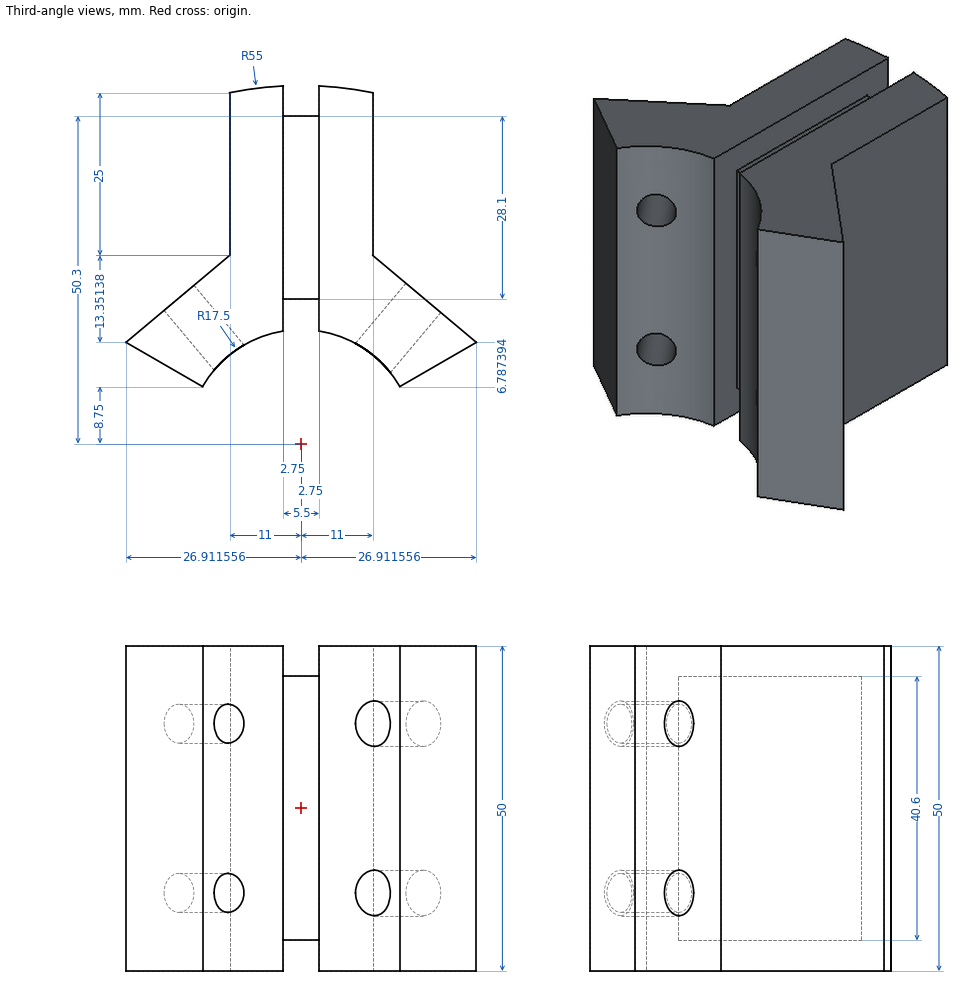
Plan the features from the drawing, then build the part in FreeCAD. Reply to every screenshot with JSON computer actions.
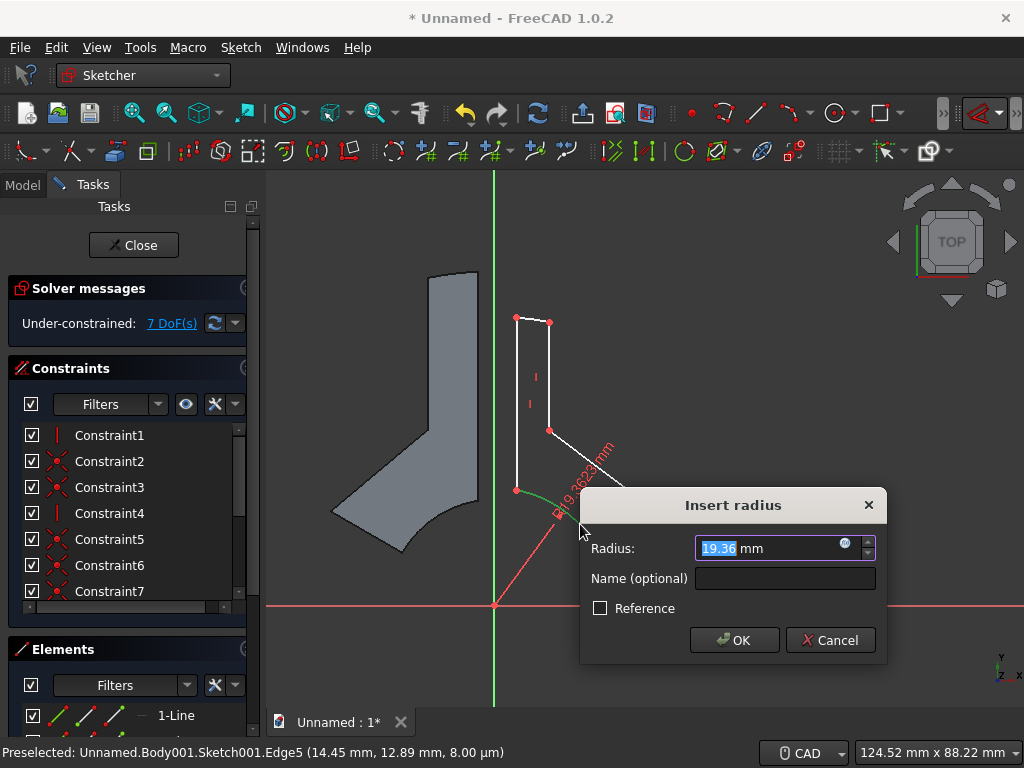
{"action": "type", "text": "17.5"}
{"action": "key", "text": "Return"}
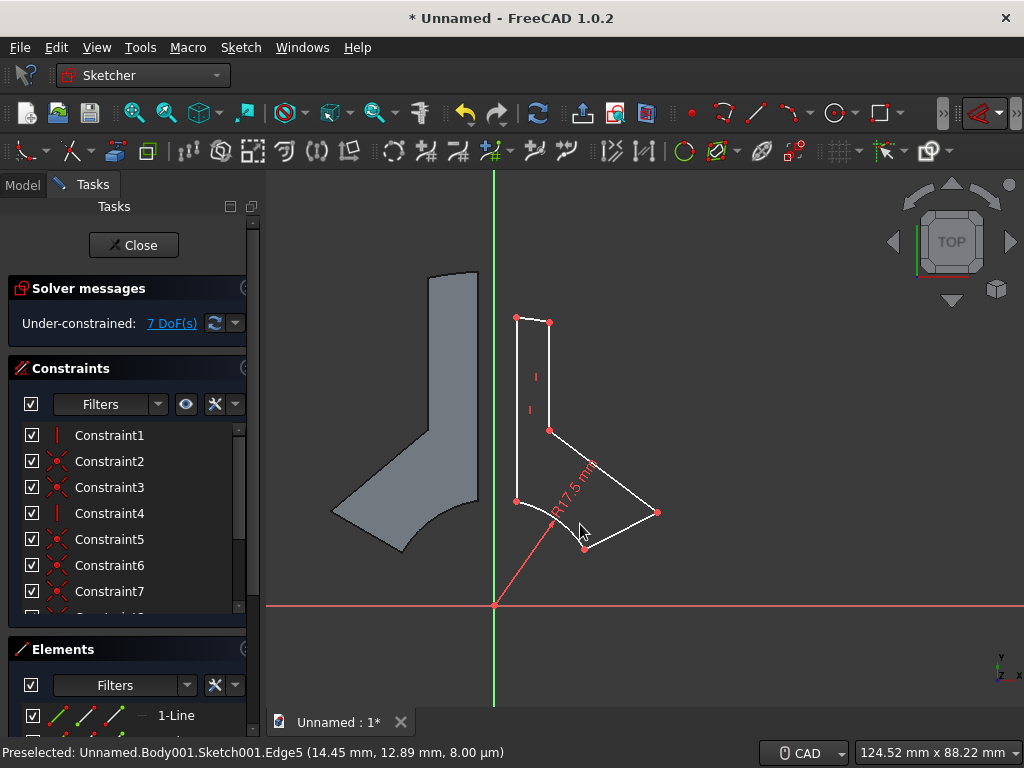
{"action": "scroll", "coordinate": [540, 320], "scroll_direction": "up", "scroll_amount": 2}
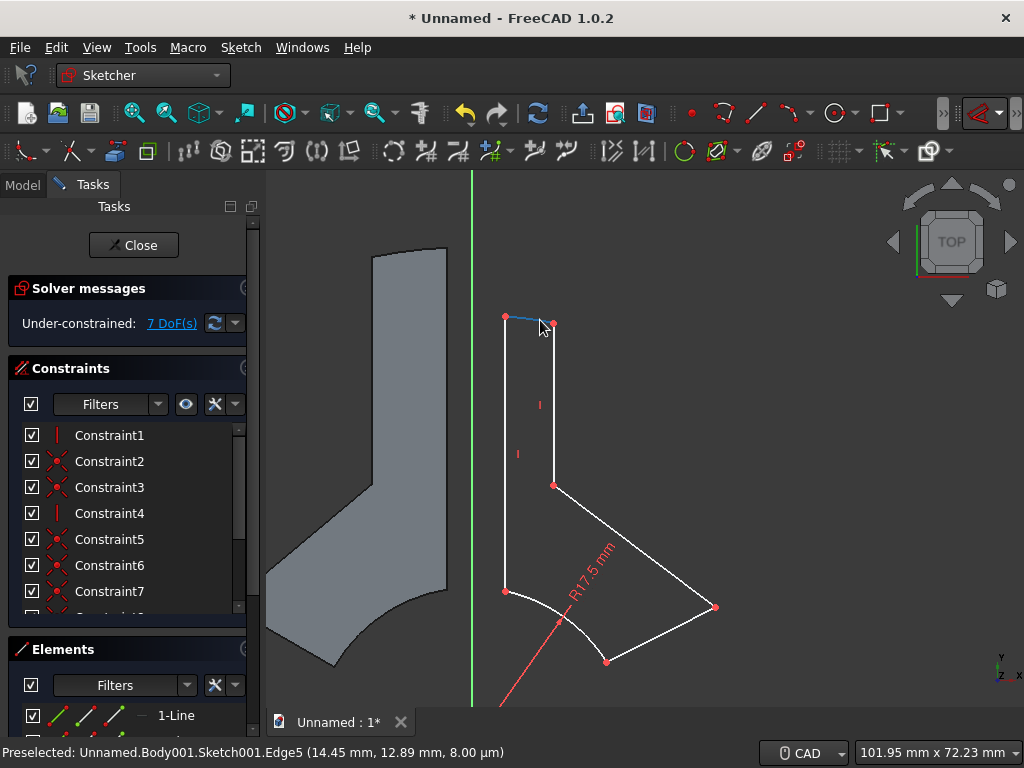
{"action": "left_click", "coordinate": [539, 320]}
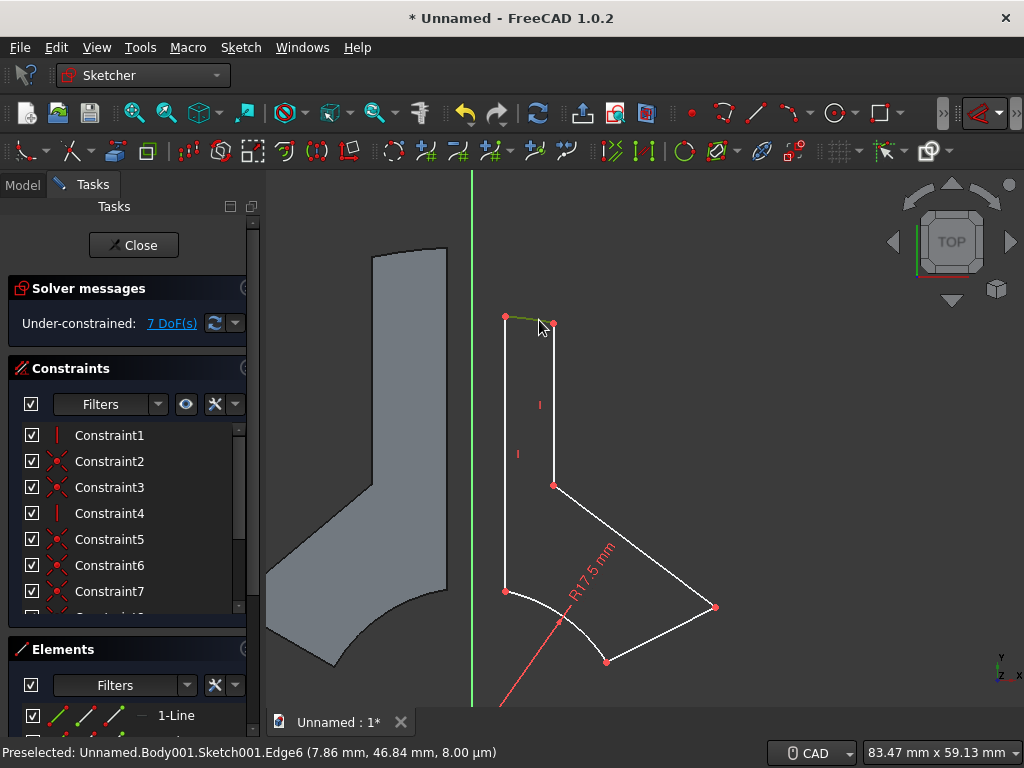
{"action": "key", "text": "k r"}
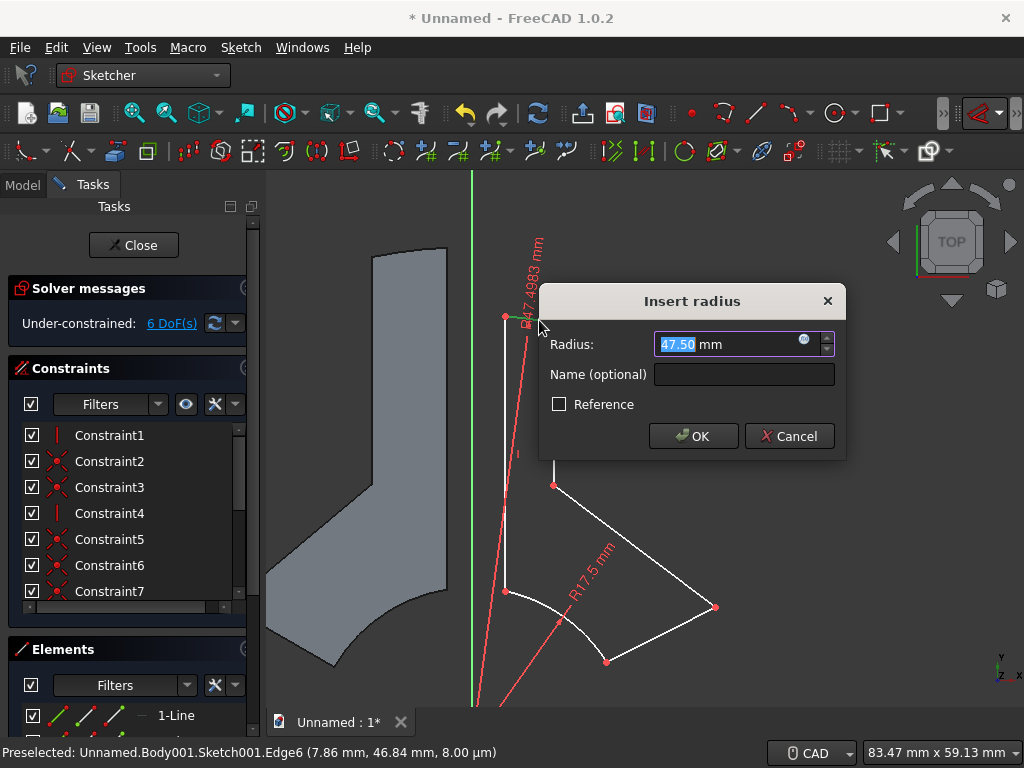
{"action": "type", "text": "55"}
{"action": "key", "text": "Return"}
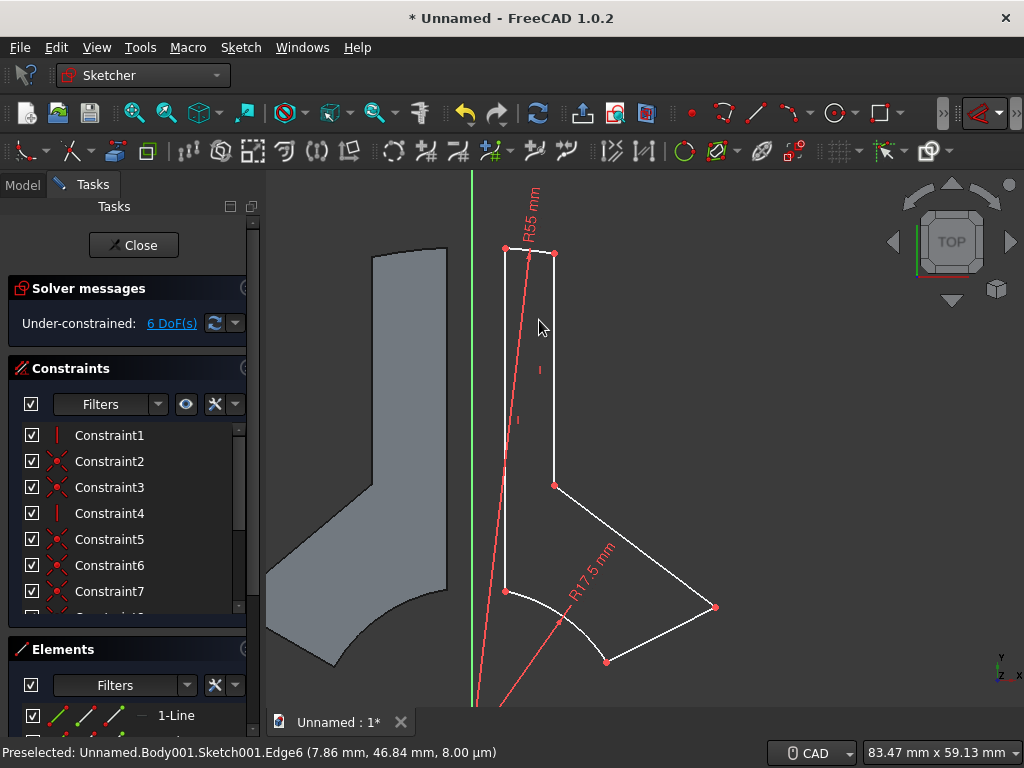
{"action": "left_click", "coordinate": [554, 416]}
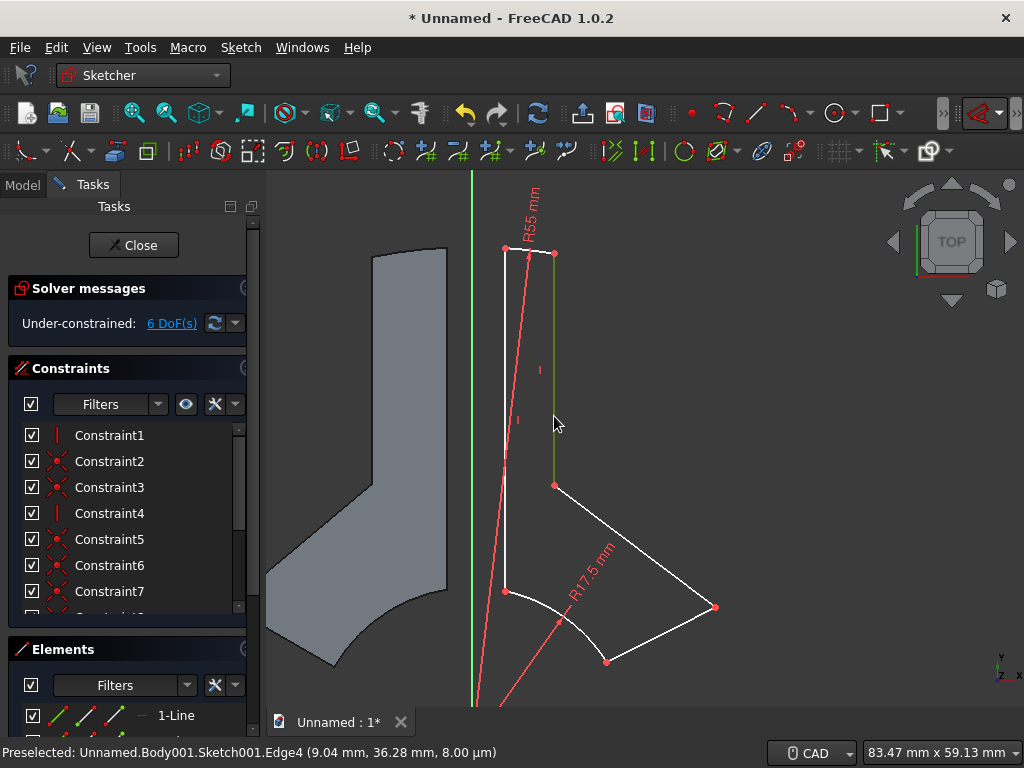
{"action": "left_click", "coordinate": [1002, 114]}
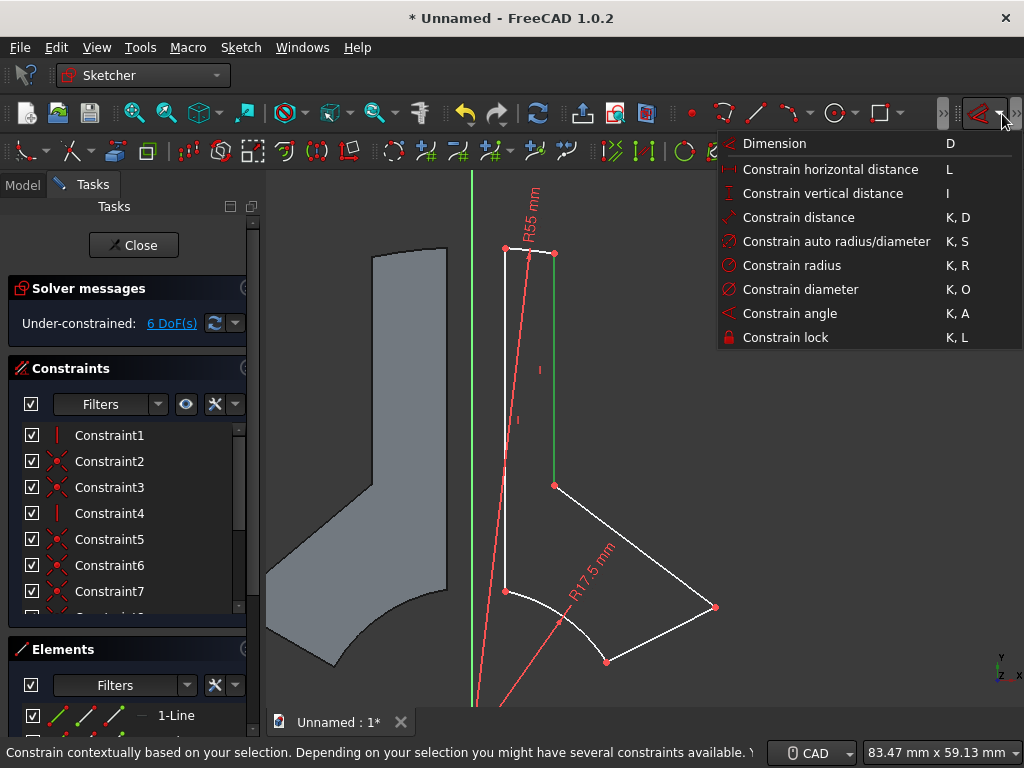
{"action": "left_click", "coordinate": [870, 193]}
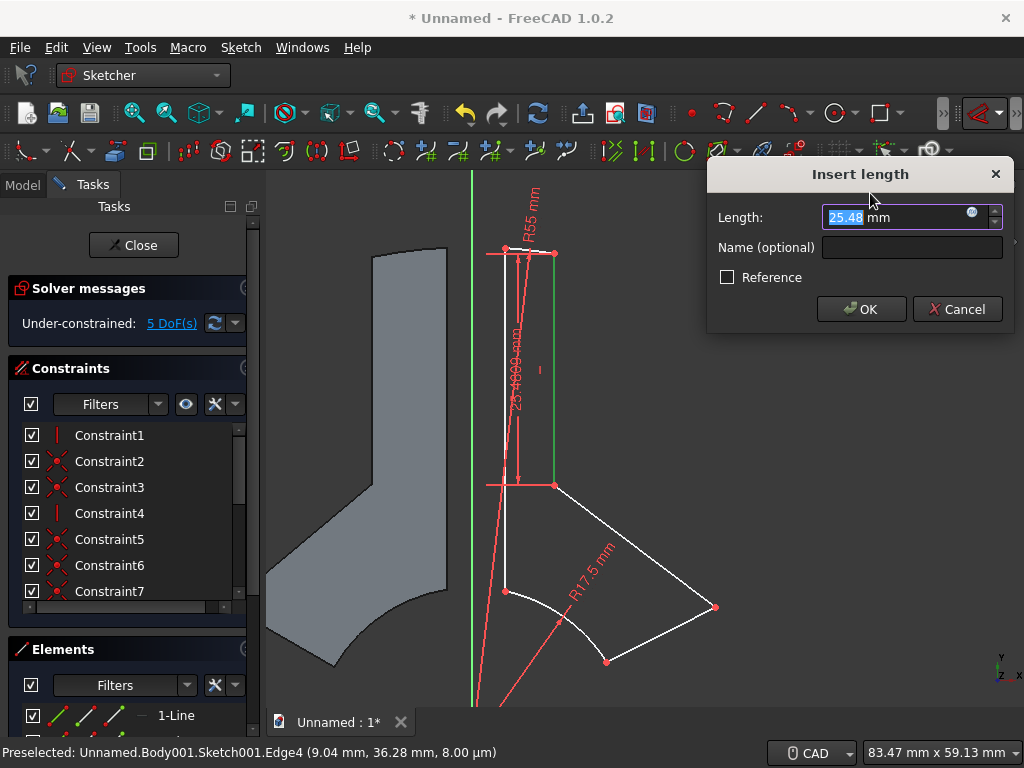
{"action": "type", "text": "25"}
{"action": "key", "text": "Return"}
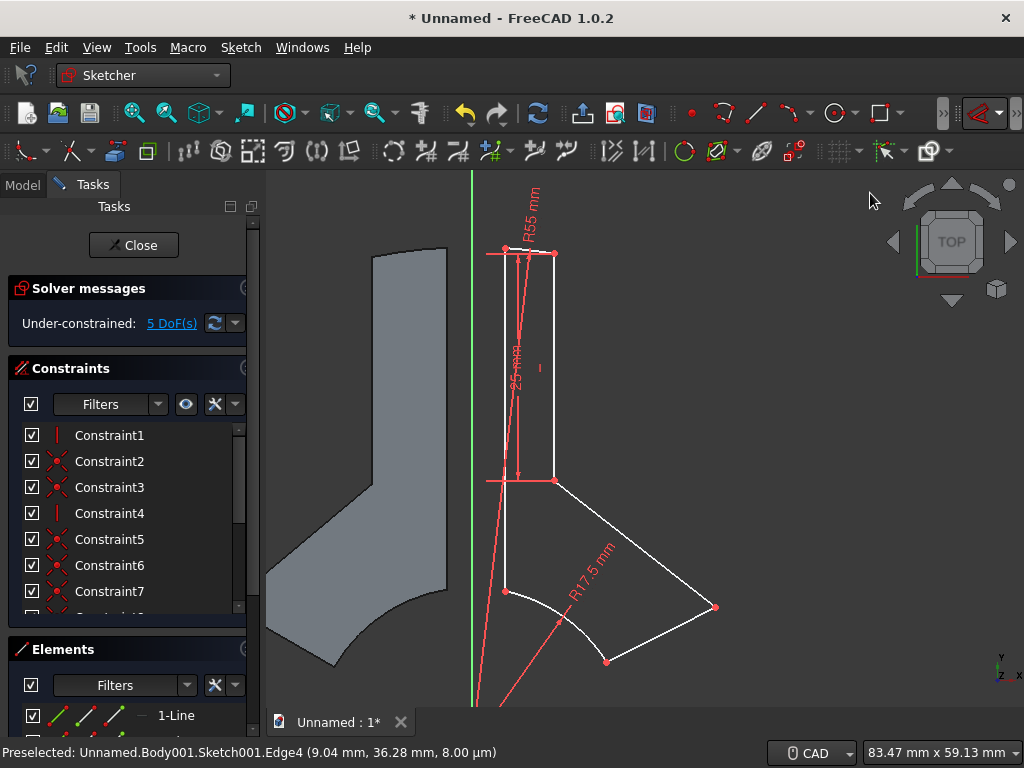
{"action": "left_click", "coordinate": [554, 481]}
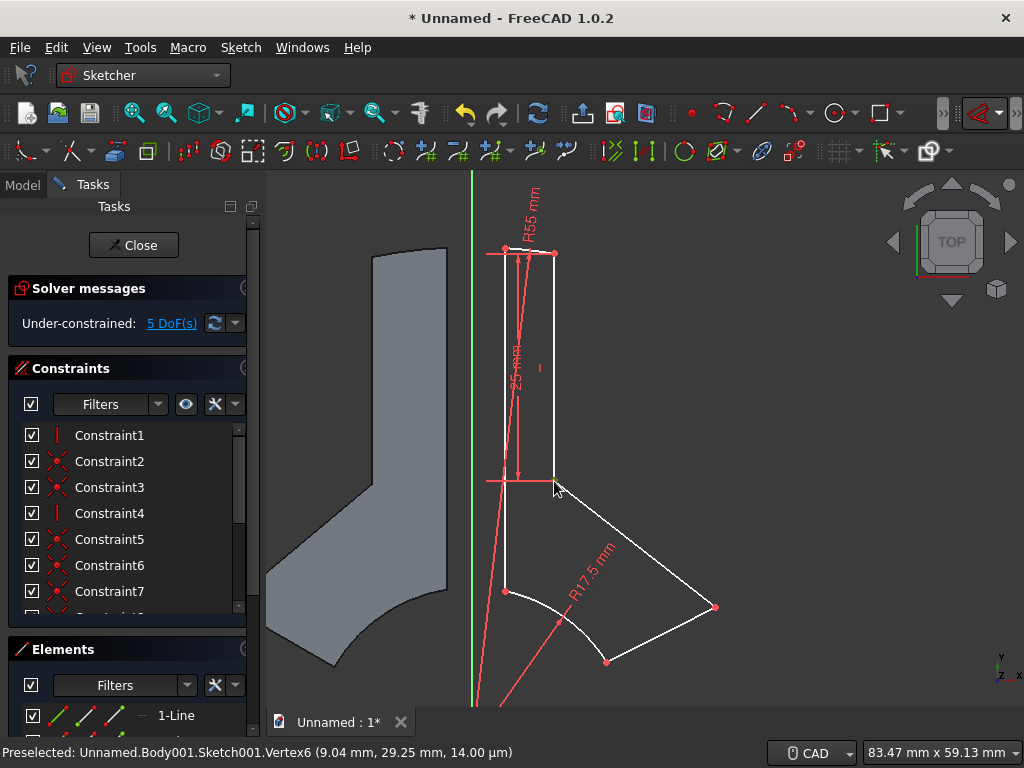
{"action": "key", "text": "l"}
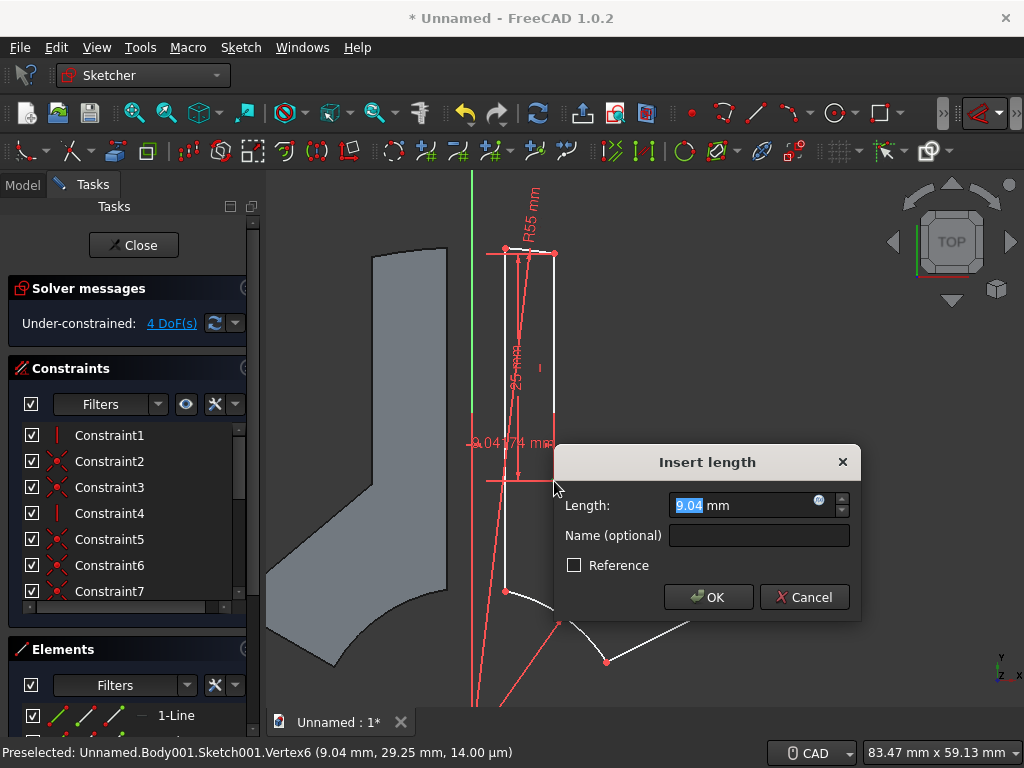
{"action": "type", "text": "11"}
{"action": "key", "text": "Return"}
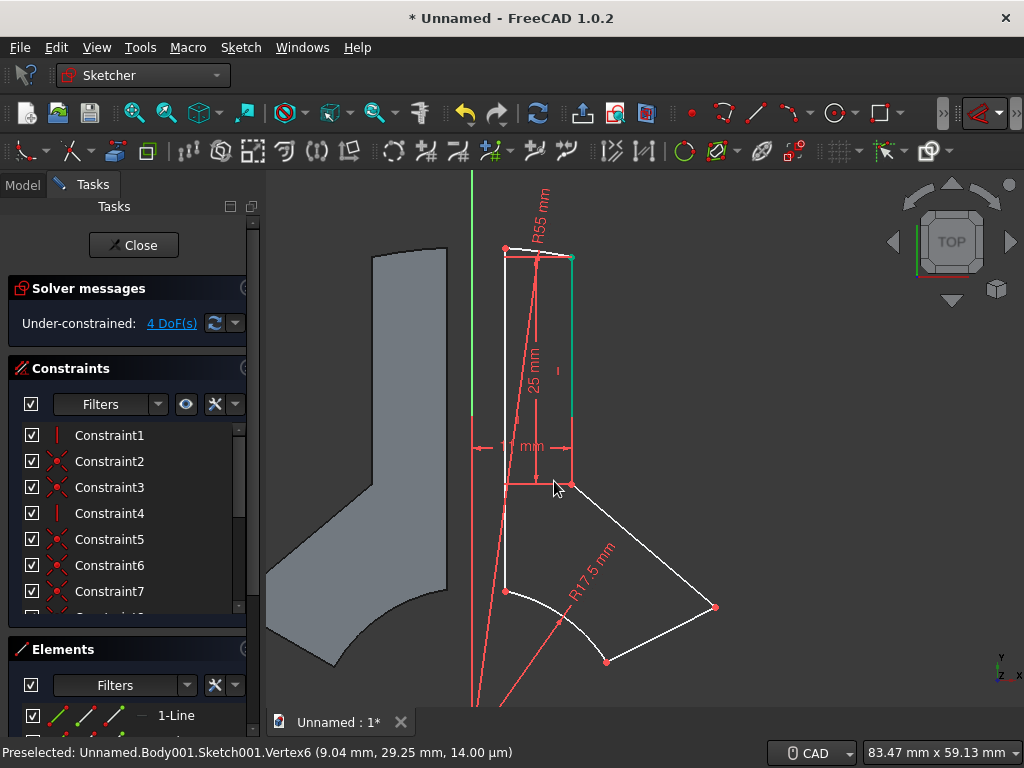
{"action": "scroll", "coordinate": [505, 248], "scroll_direction": "up", "scroll_amount": 3}